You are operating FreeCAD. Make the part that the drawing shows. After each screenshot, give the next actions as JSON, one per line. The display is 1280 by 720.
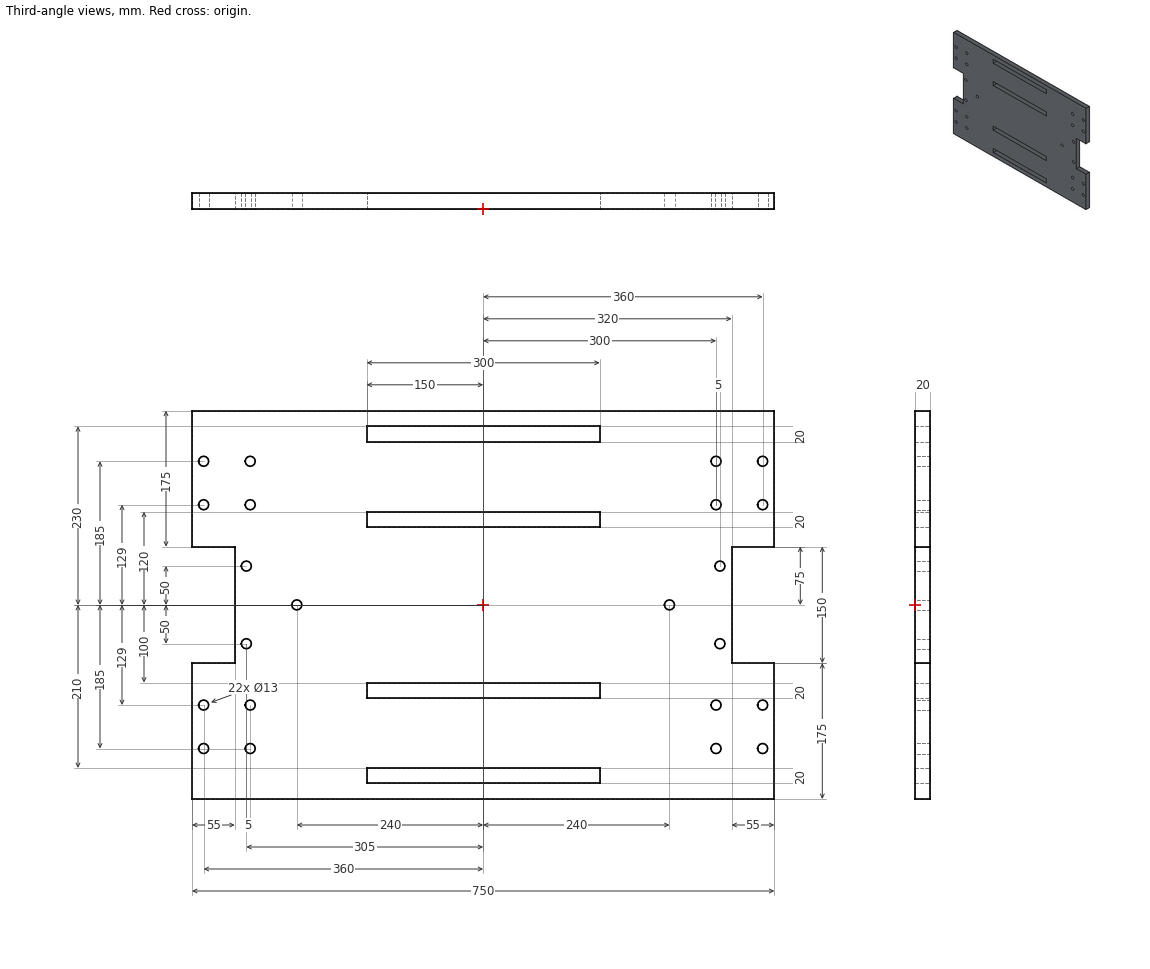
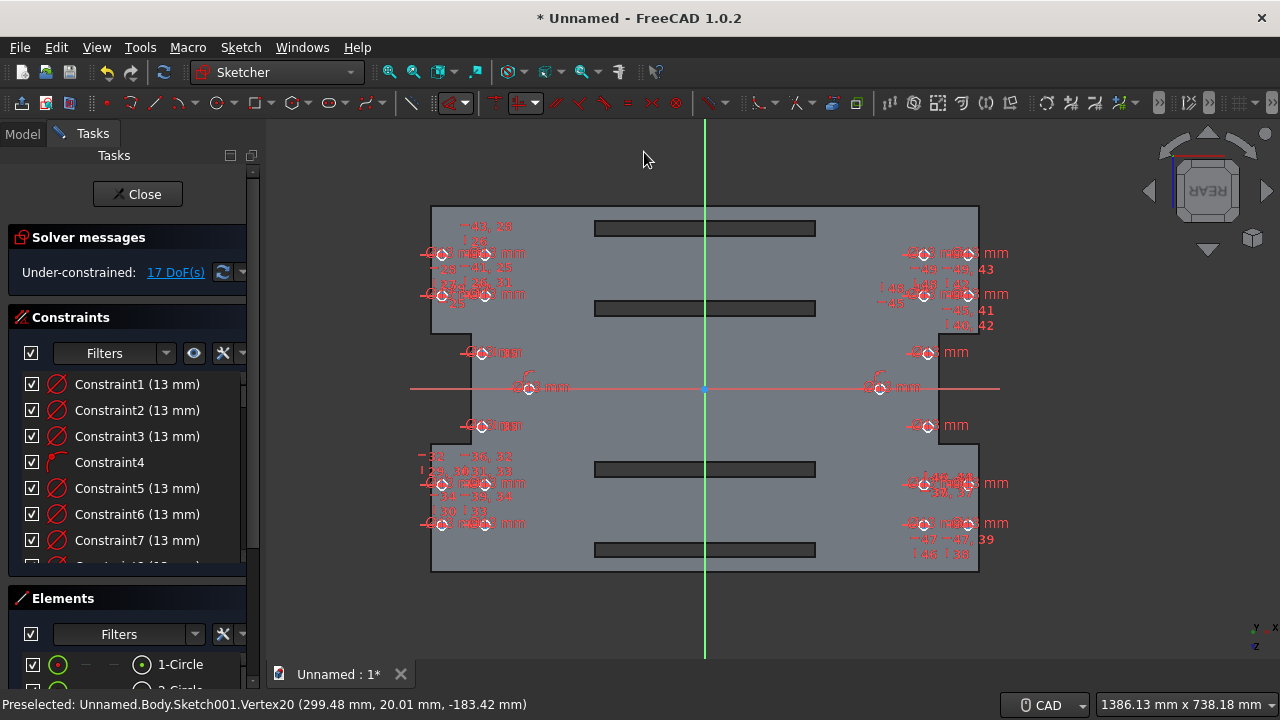
{"action": "left_click", "coordinate": [928, 427]}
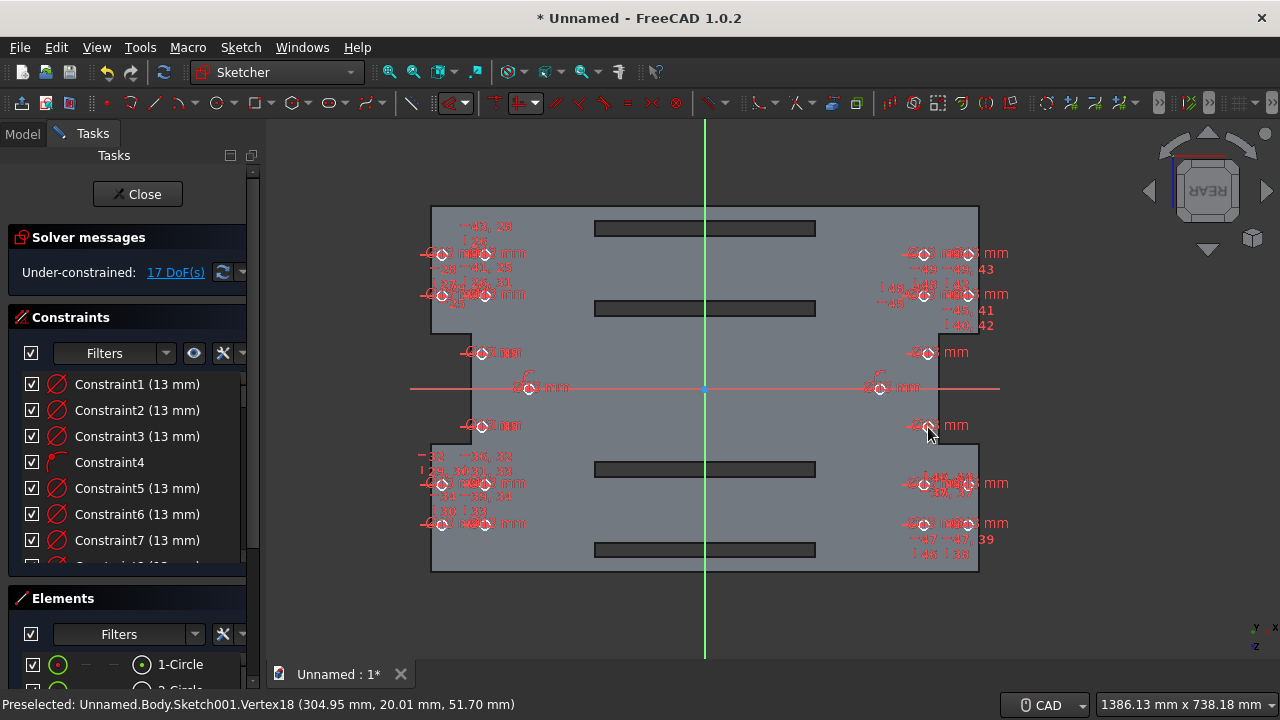
{"action": "left_click", "coordinate": [928, 354]}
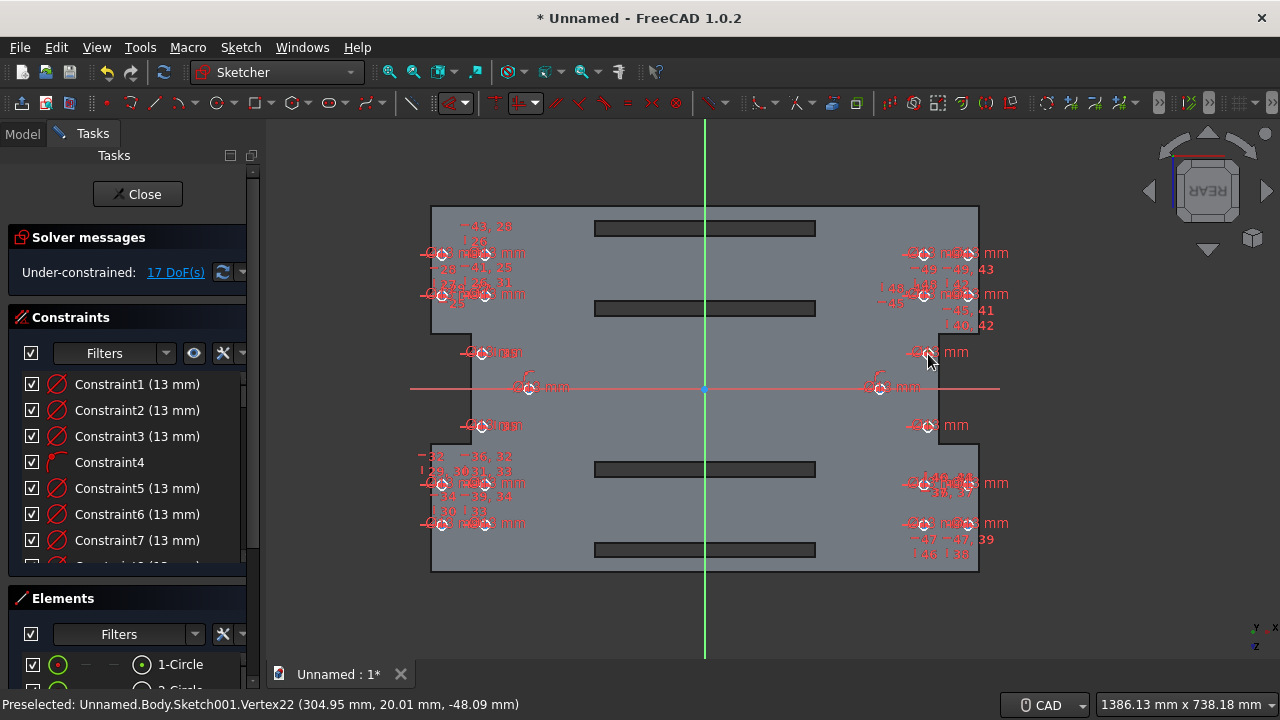
{"action": "key", "text": "v"}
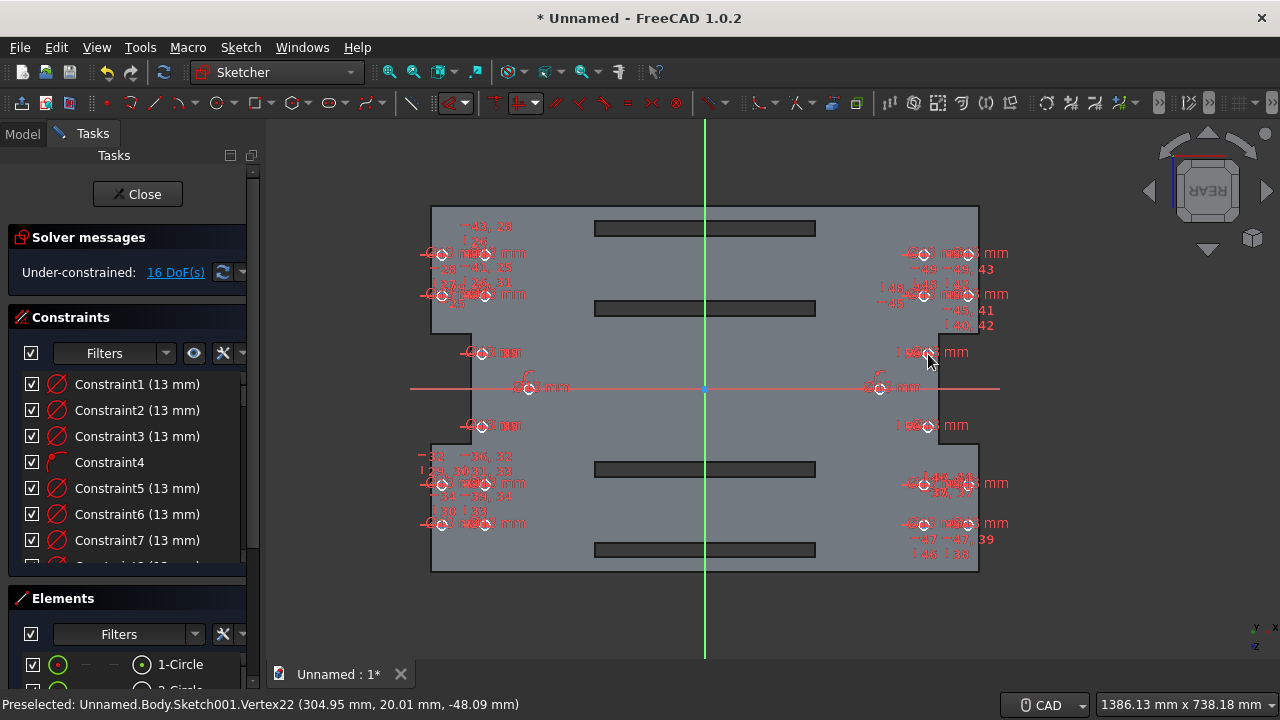
{"action": "left_click", "coordinate": [482, 354]}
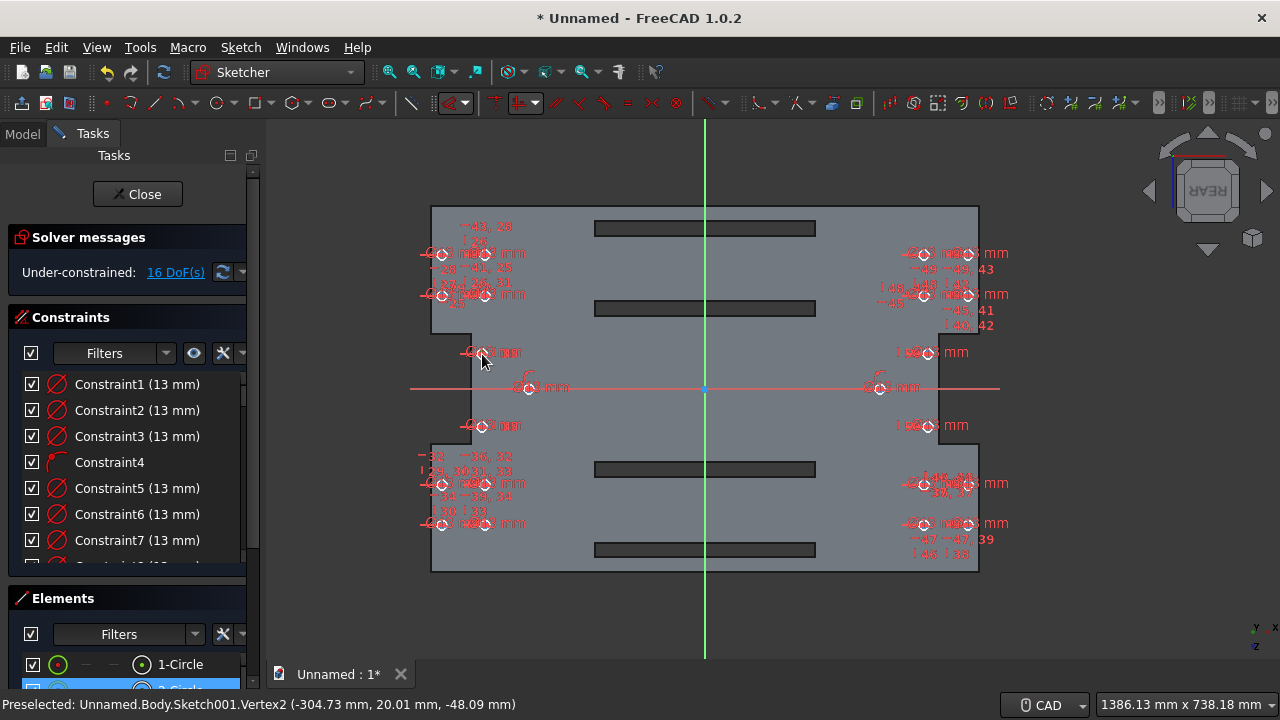
{"action": "left_click", "coordinate": [468, 104]}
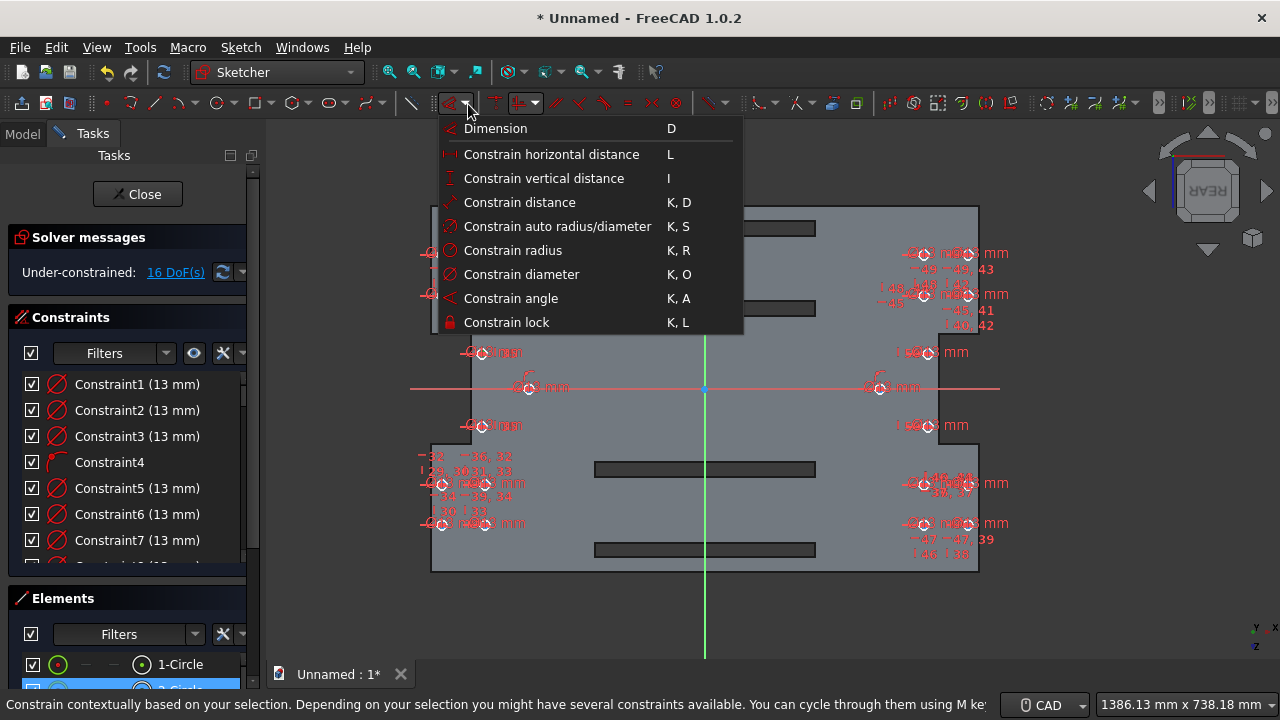
{"action": "left_click", "coordinate": [591, 178]}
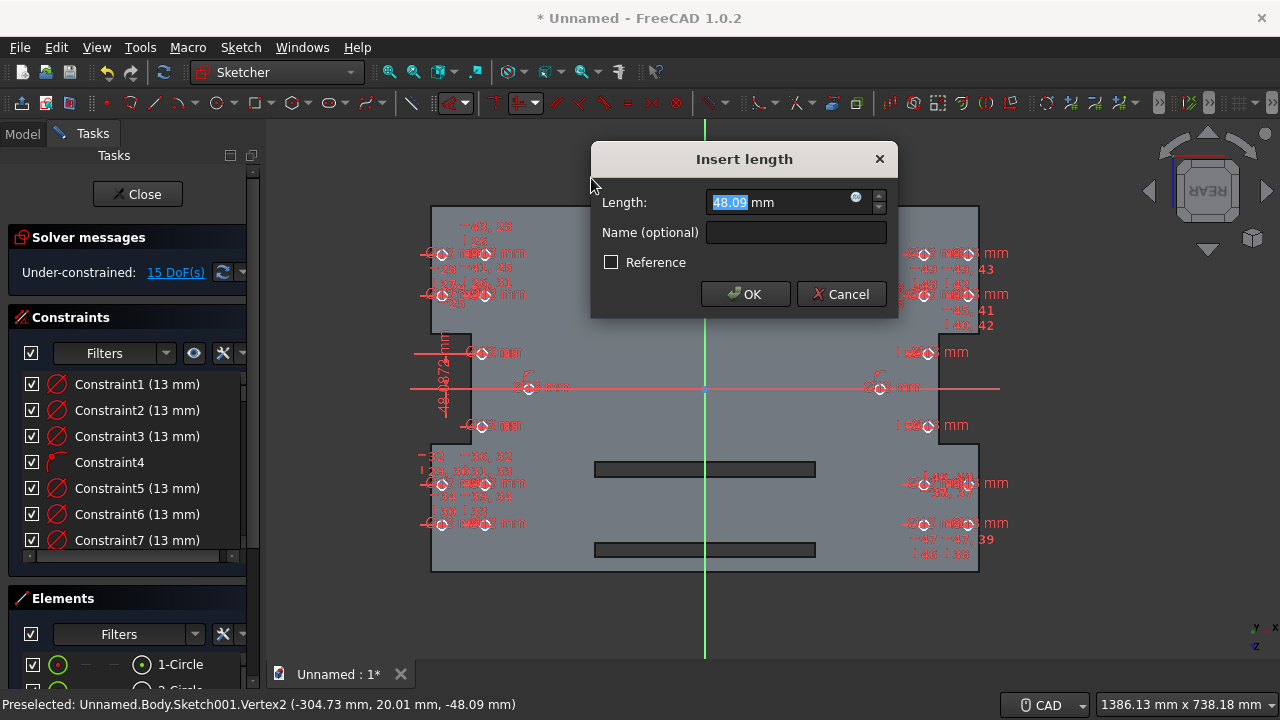
{"action": "type", "text": "50"}
{"action": "key", "text": "Return"}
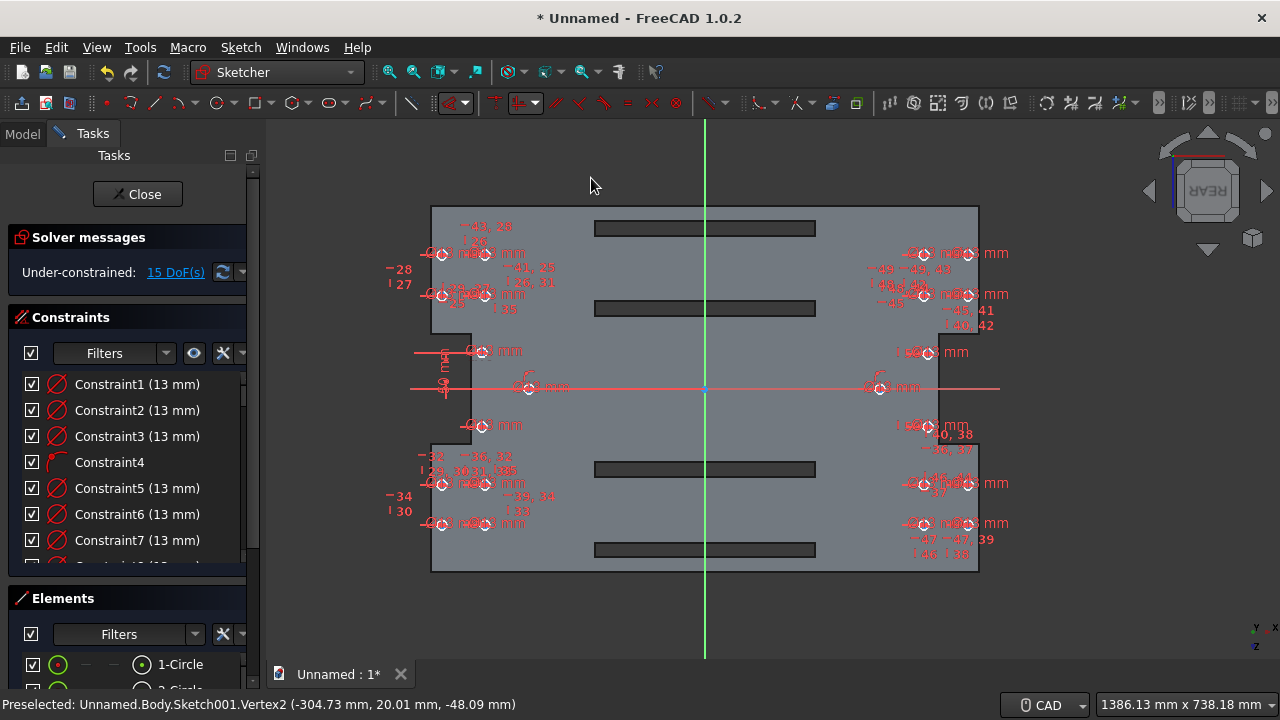
{"action": "left_click", "coordinate": [482, 427]}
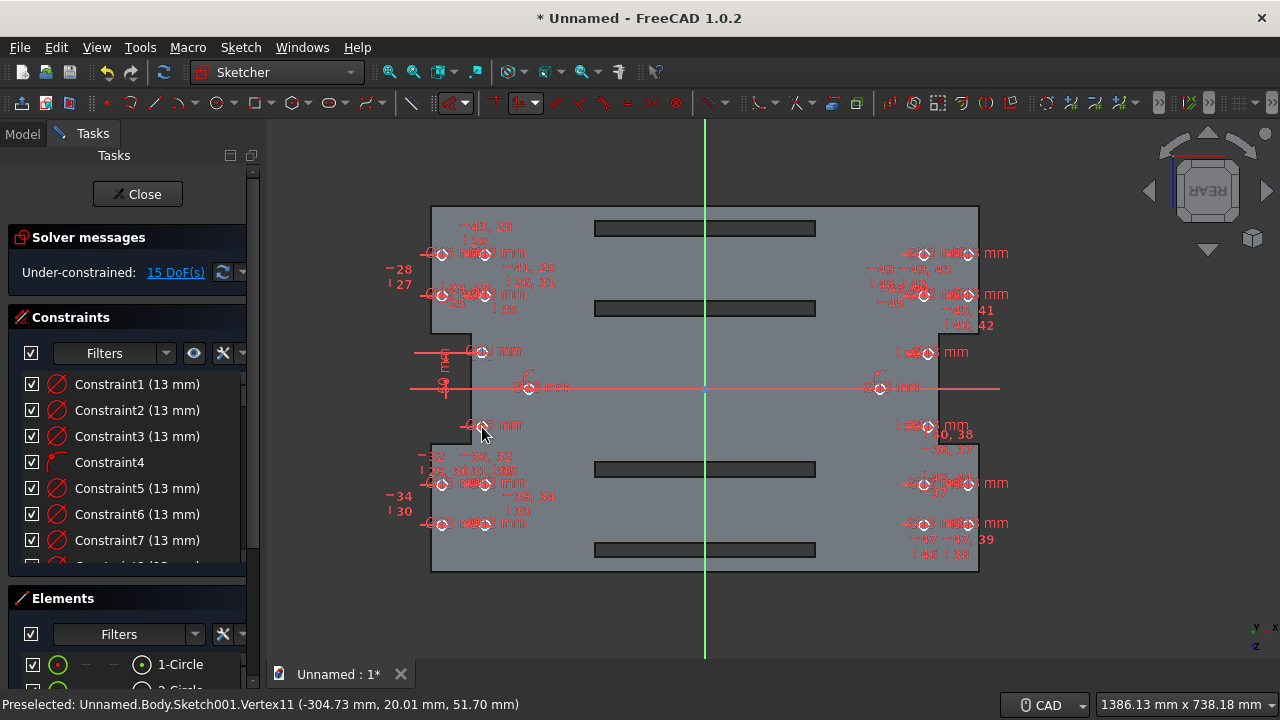
{"action": "key", "text": "i"}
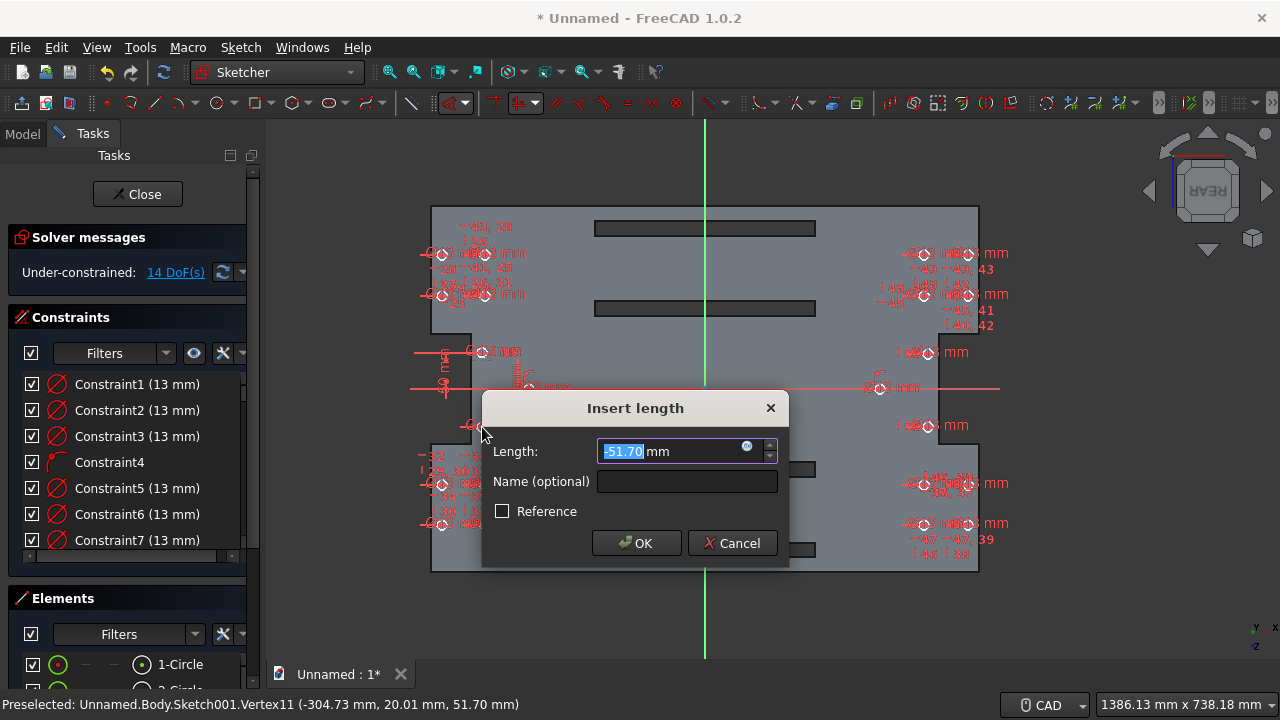
{"action": "type", "text": "-50"}
{"action": "key", "text": "Return"}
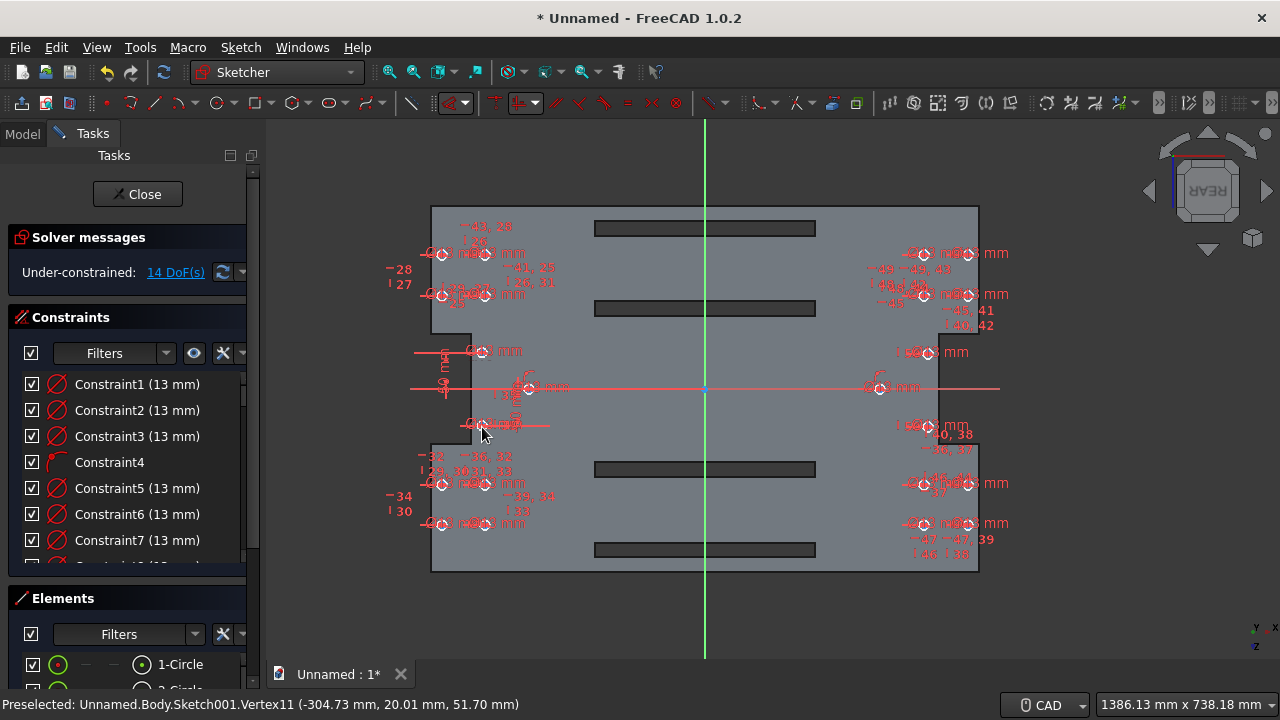
{"action": "left_click", "coordinate": [928, 427]}